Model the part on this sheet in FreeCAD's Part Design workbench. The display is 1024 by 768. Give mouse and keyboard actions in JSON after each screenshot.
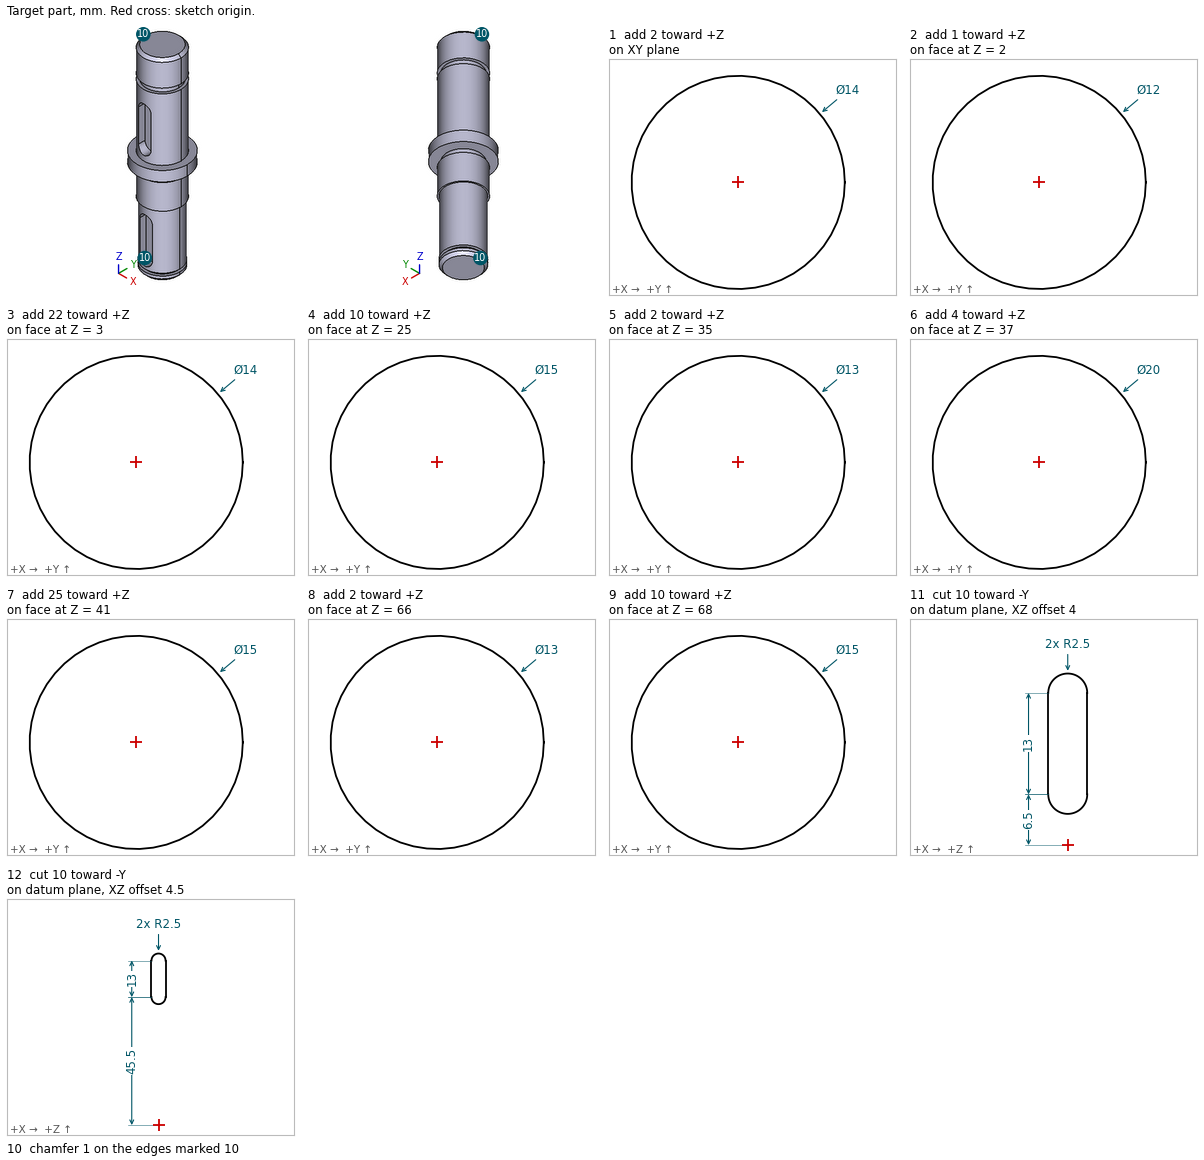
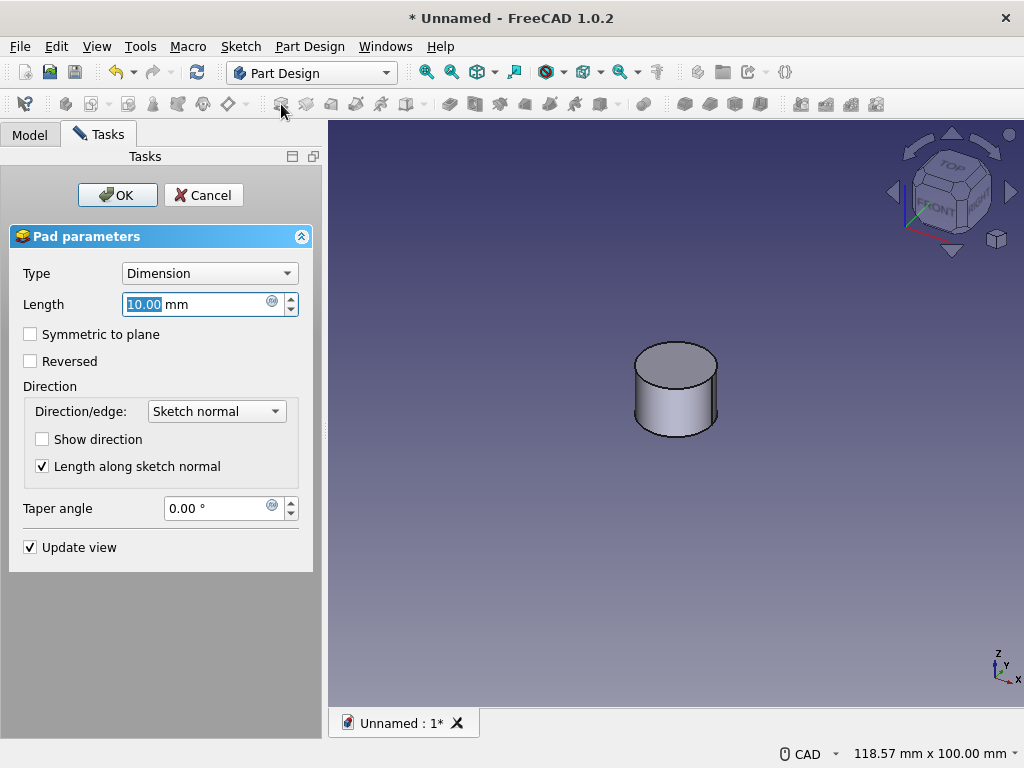
{"action": "type", "text": "2"}
{"action": "key", "text": "Tab"}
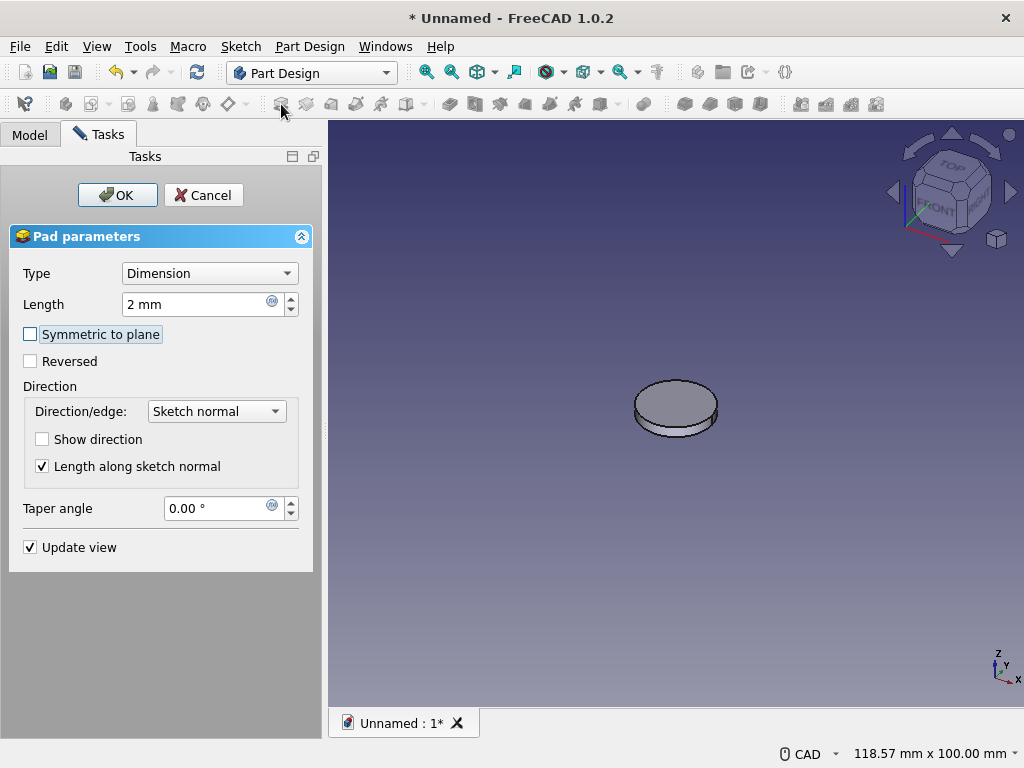
{"action": "left_click", "coordinate": [118, 195]}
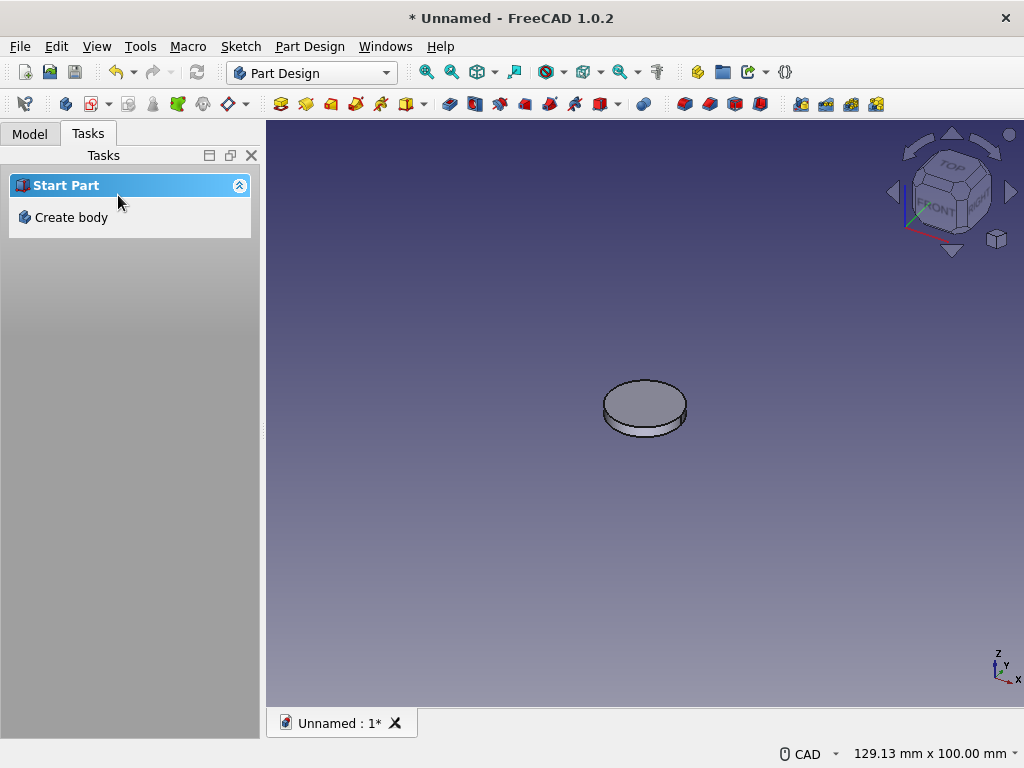
{"action": "left_click", "coordinate": [427, 72]}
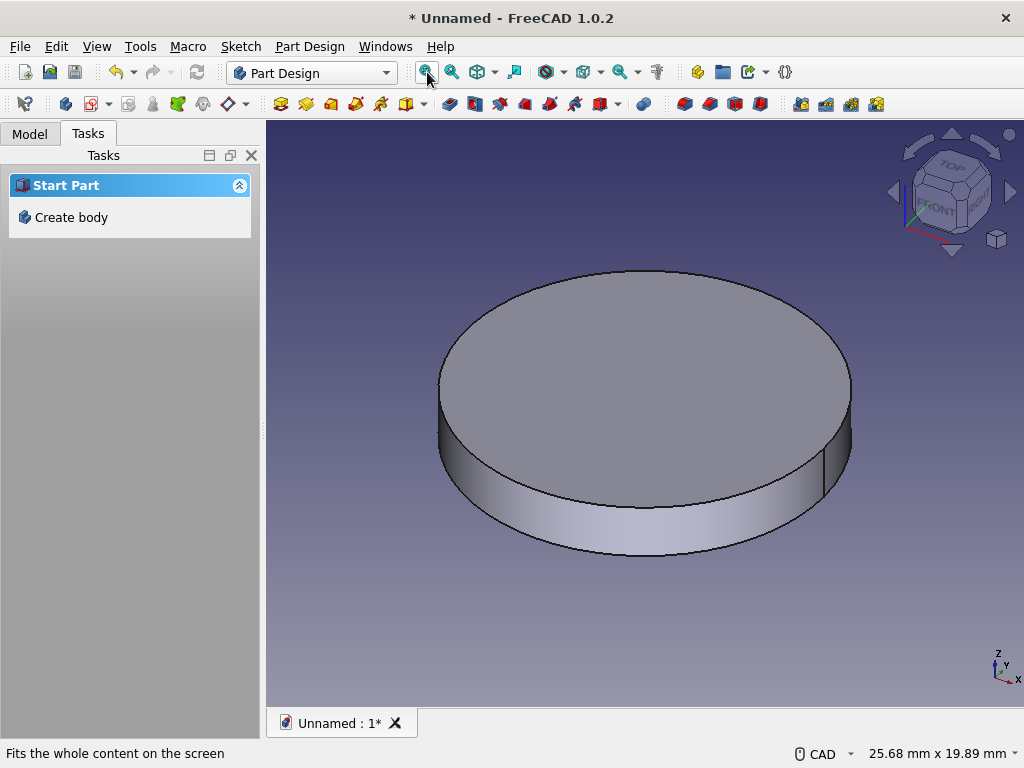
{"action": "left_click", "coordinate": [645, 388]}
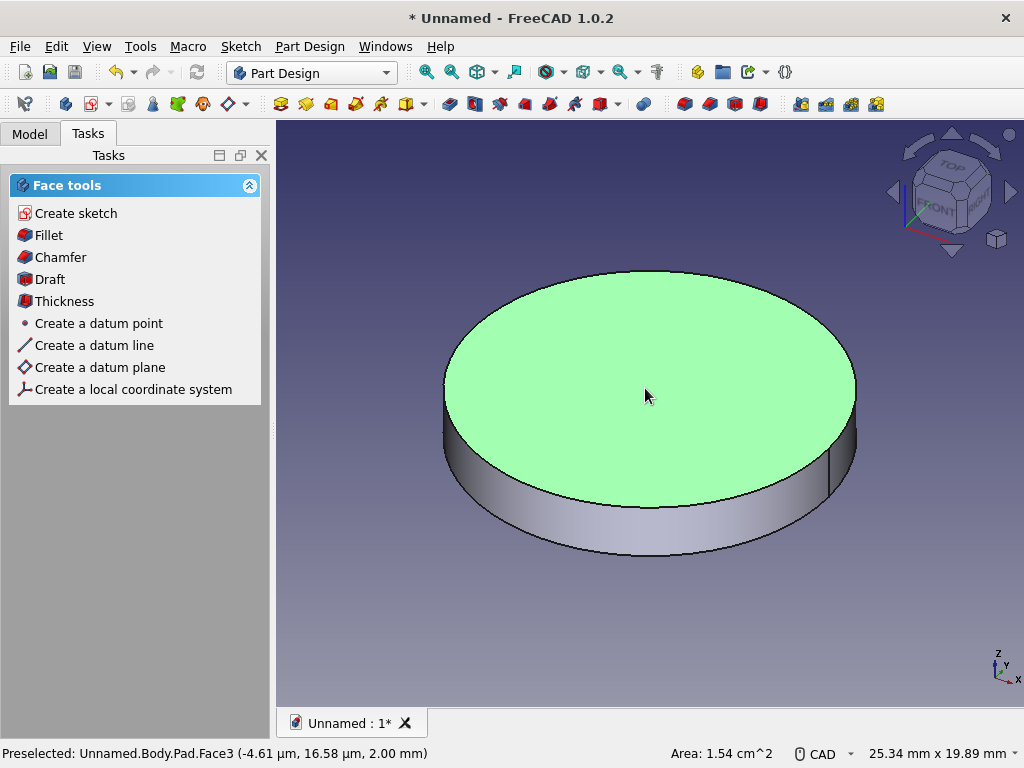
{"action": "left_click", "coordinate": [90, 104]}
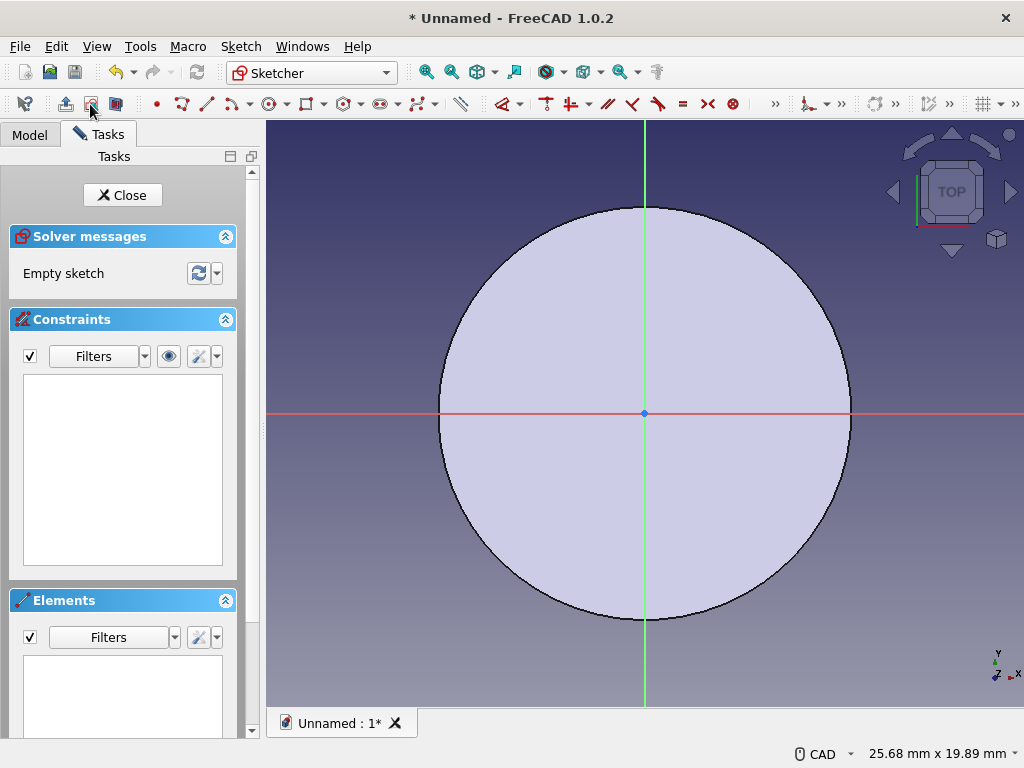
{"action": "left_click", "coordinate": [268, 104]}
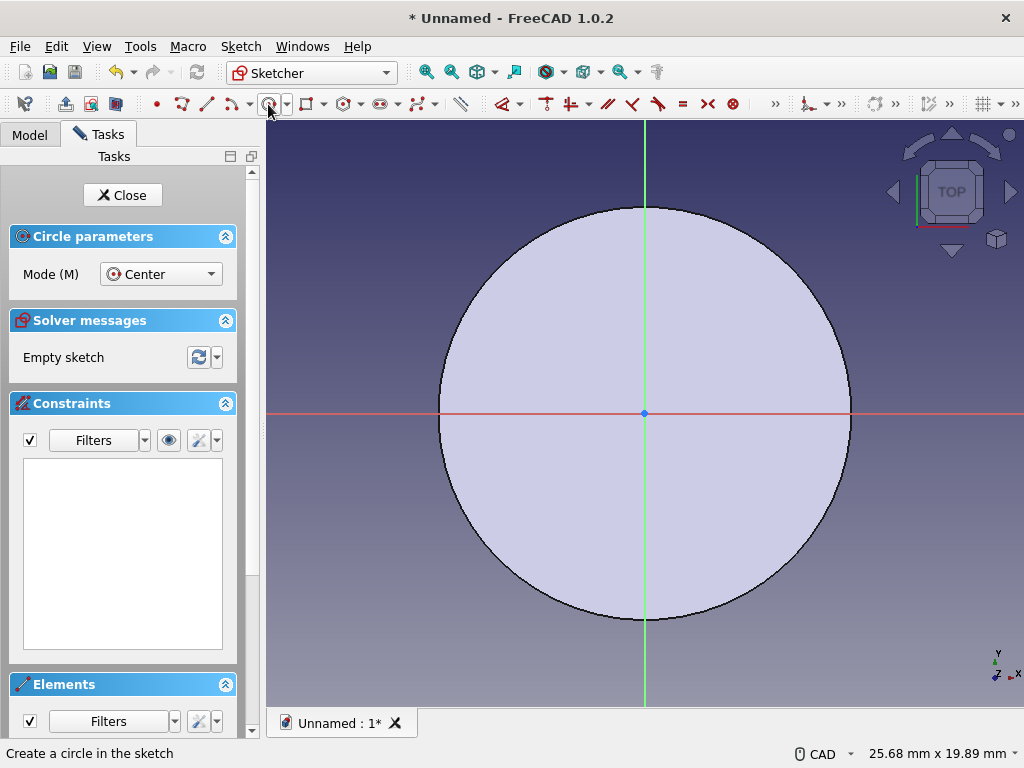
{"action": "left_click", "coordinate": [645, 414]}
{"action": "left_click", "coordinate": [770, 288]}
{"action": "key", "text": "Escape"}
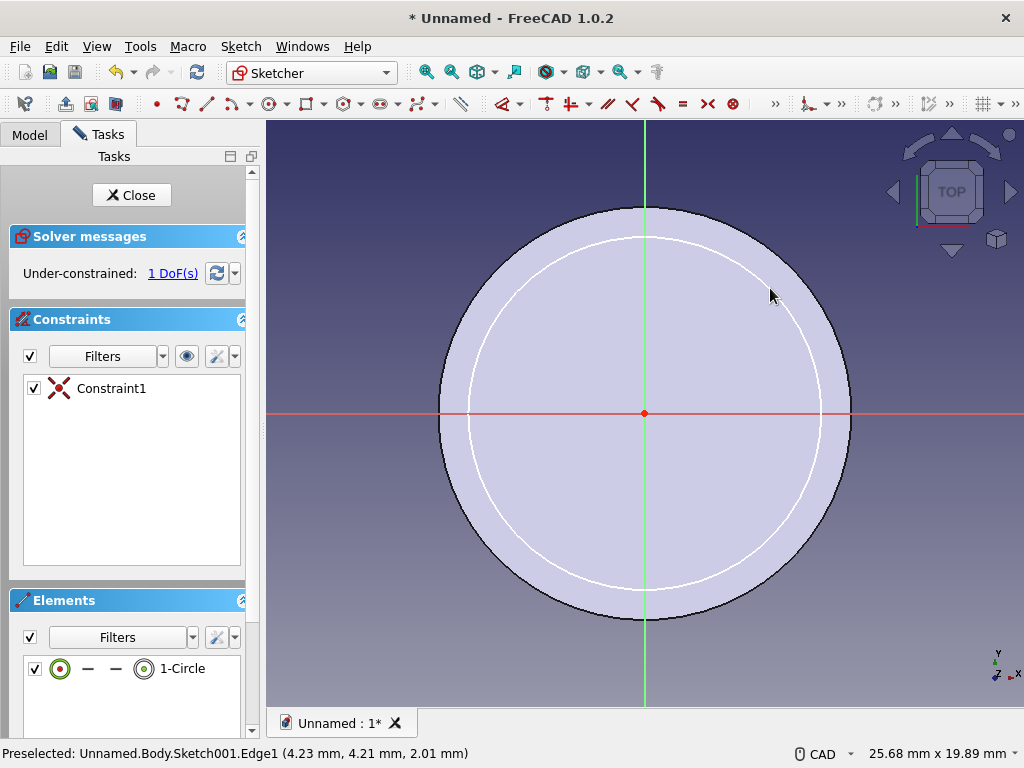
{"action": "left_click", "coordinate": [502, 104]}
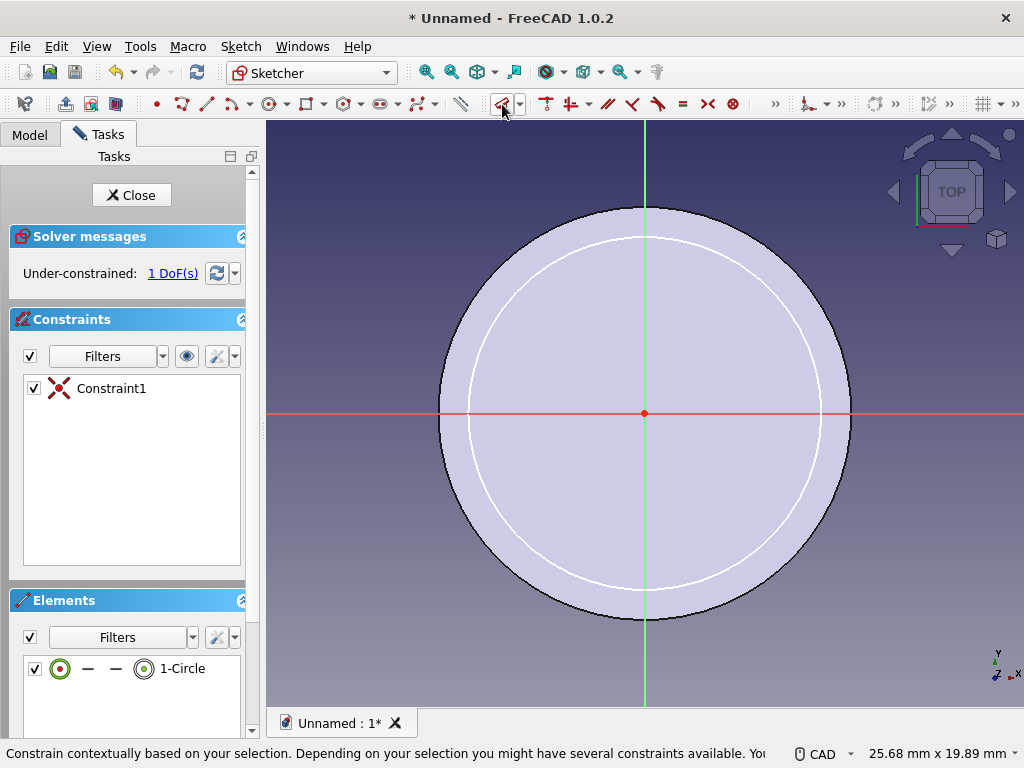
{"action": "left_click", "coordinate": [769, 288]}
{"action": "left_click", "coordinate": [792, 265]}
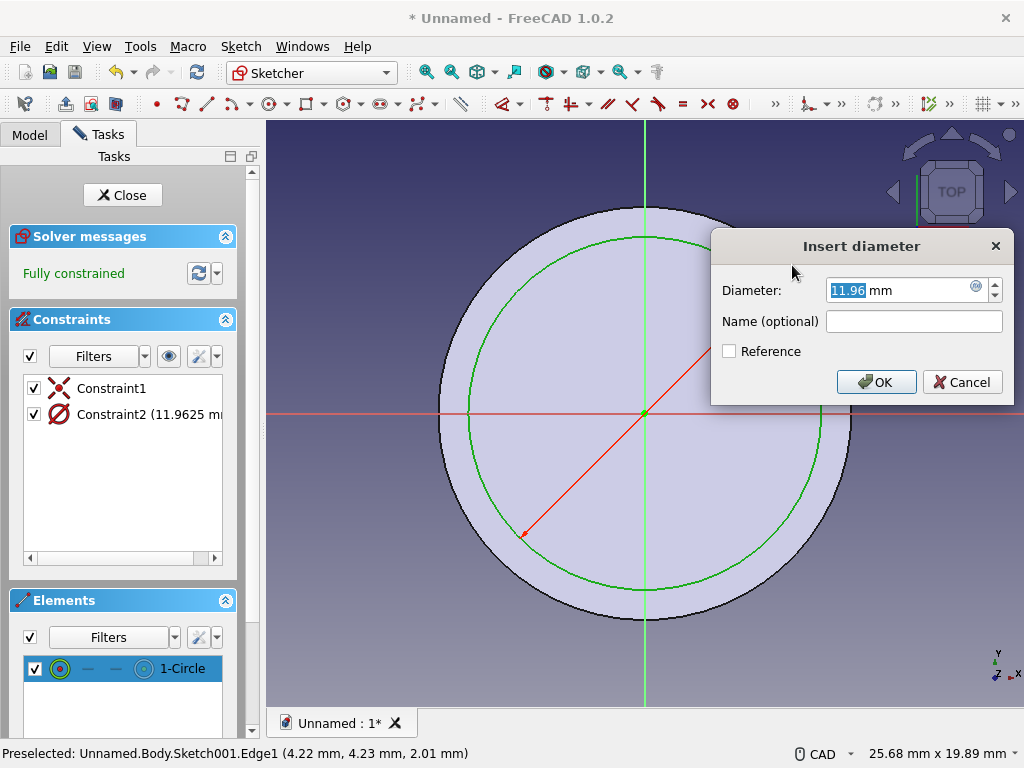
{"action": "type", "text": "12"}
{"action": "key", "text": "Return"}
{"action": "key", "text": "Escape"}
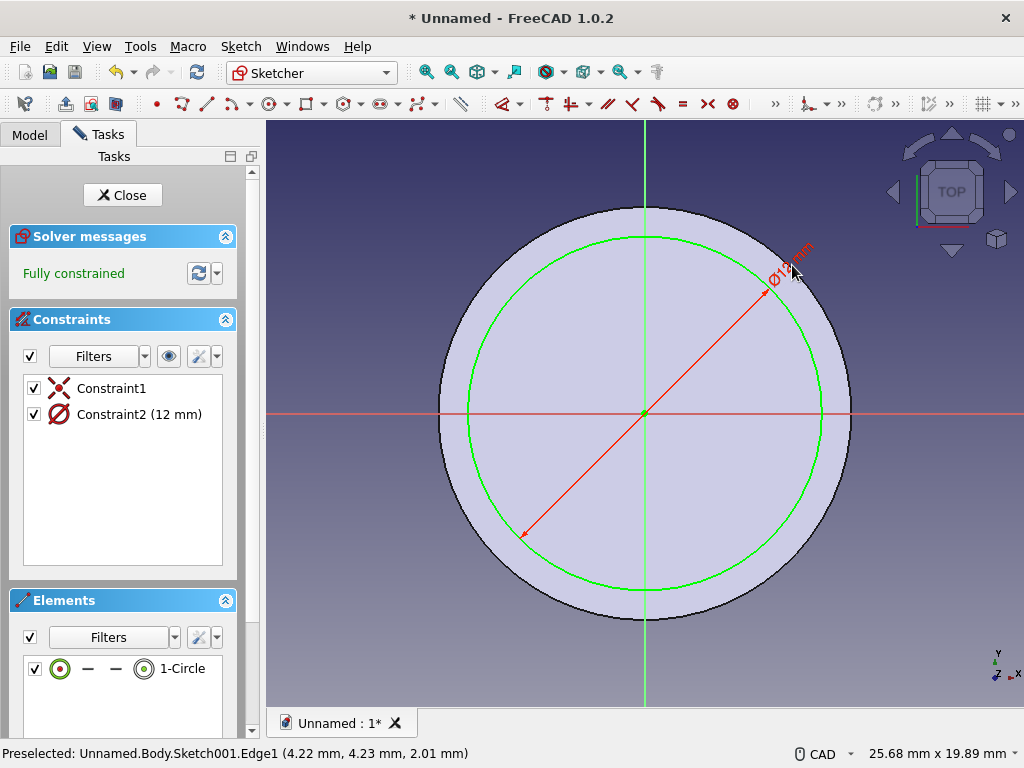
{"action": "left_click", "coordinate": [123, 195]}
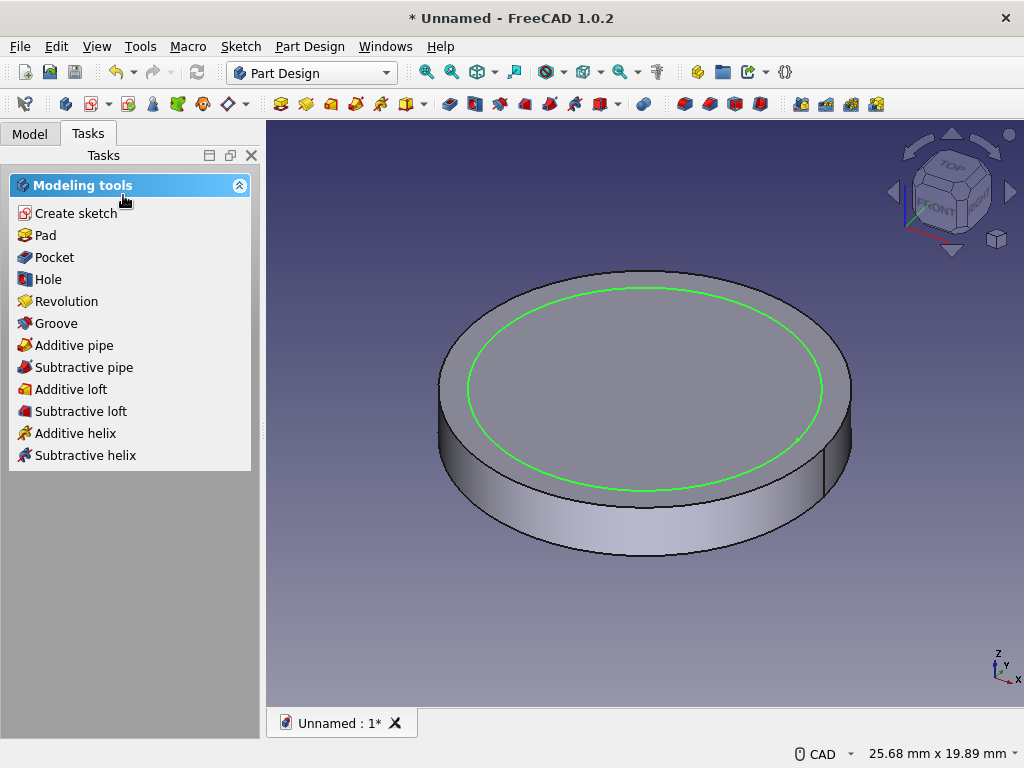
{"action": "left_click", "coordinate": [281, 104]}